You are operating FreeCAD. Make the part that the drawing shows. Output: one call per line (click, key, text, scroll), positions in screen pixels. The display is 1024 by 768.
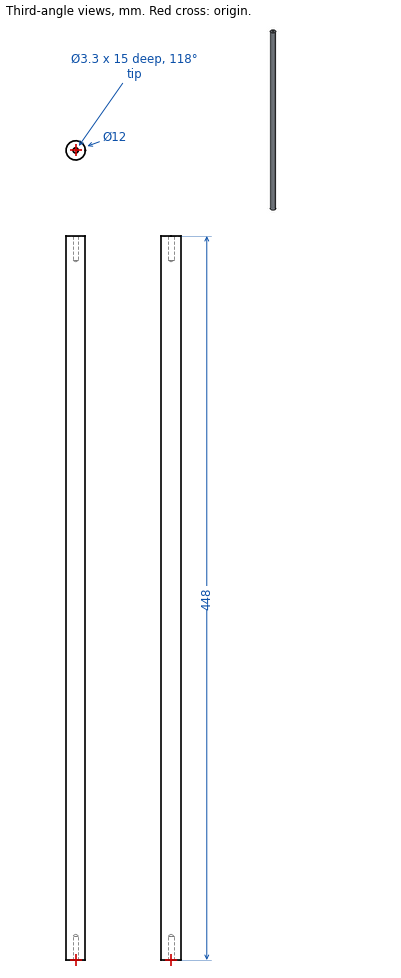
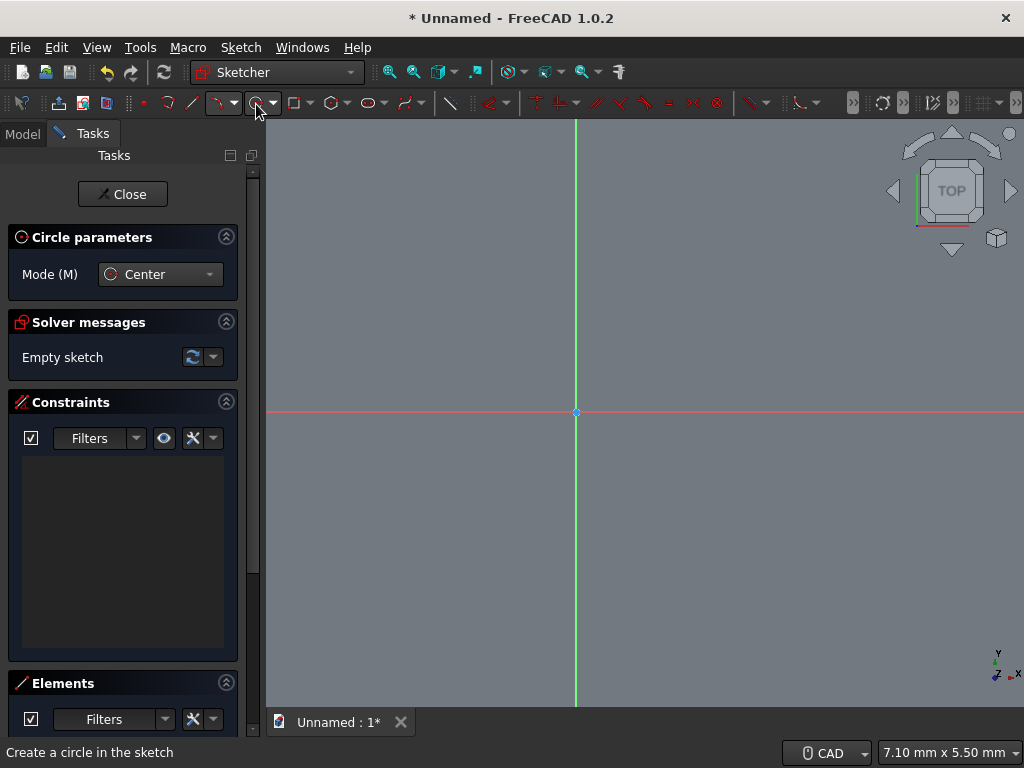
click(576, 412)
move(701, 288)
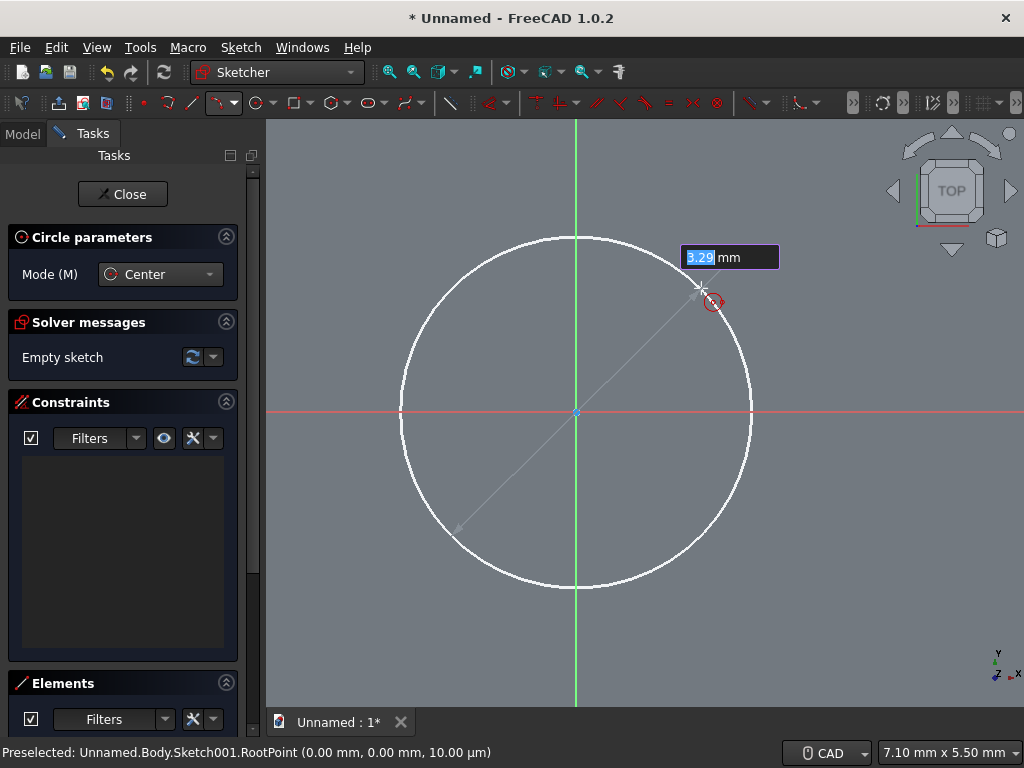
text(3.3)
key(Return)
key(Escape)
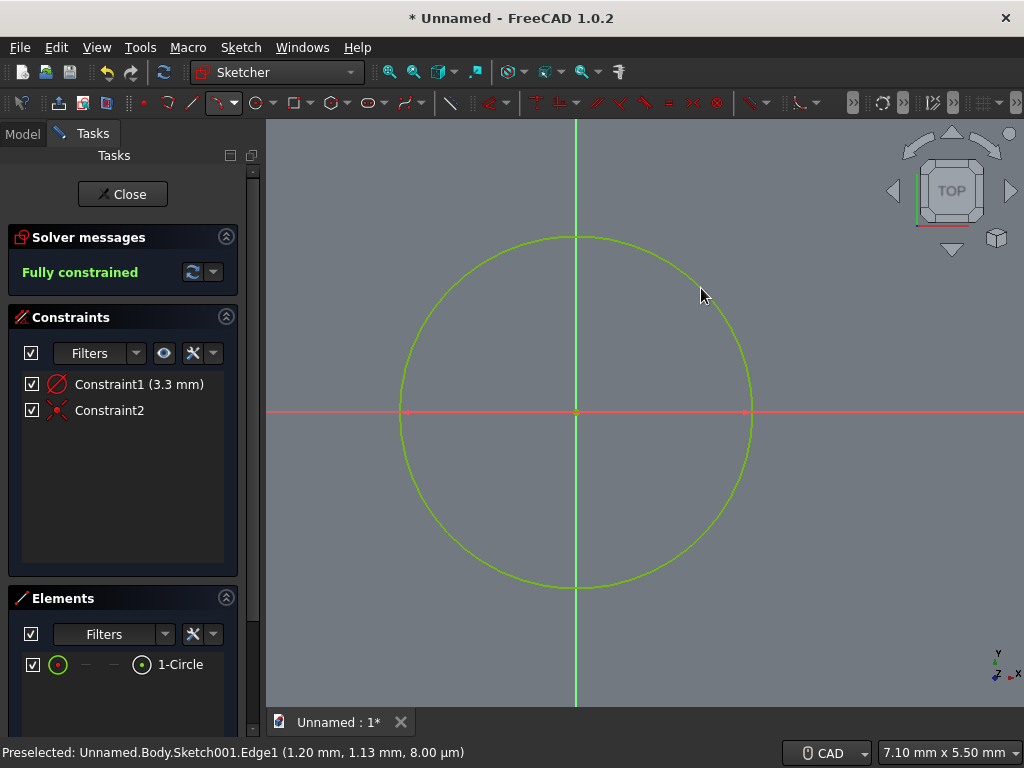
click(123, 194)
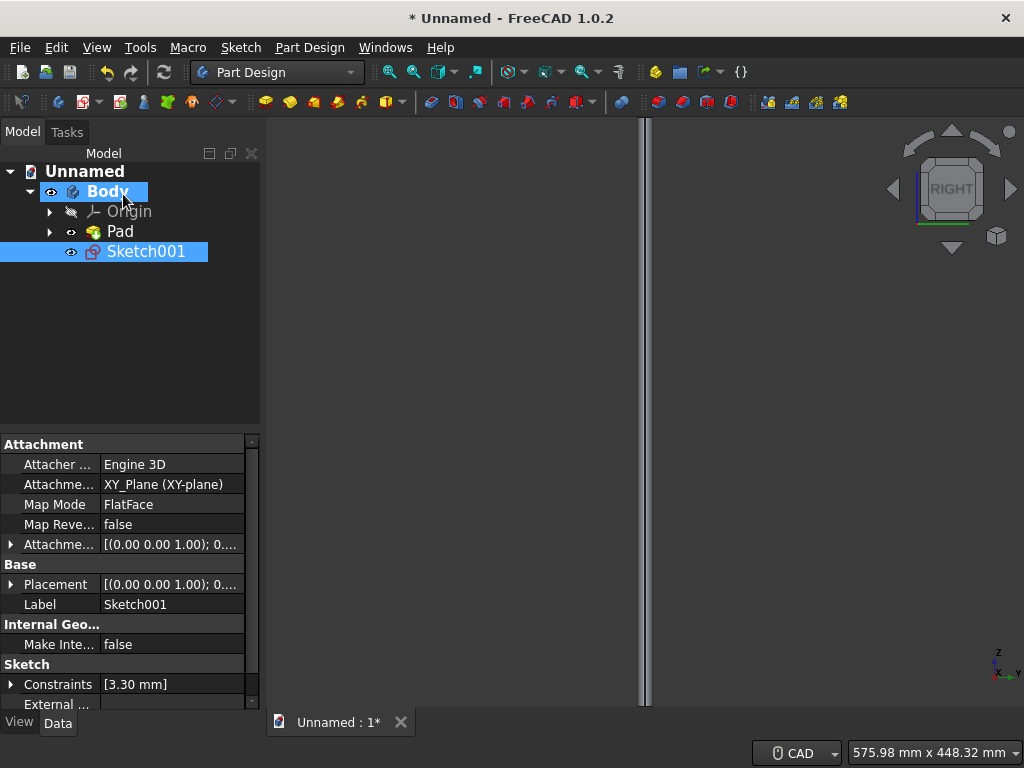
click(456, 102)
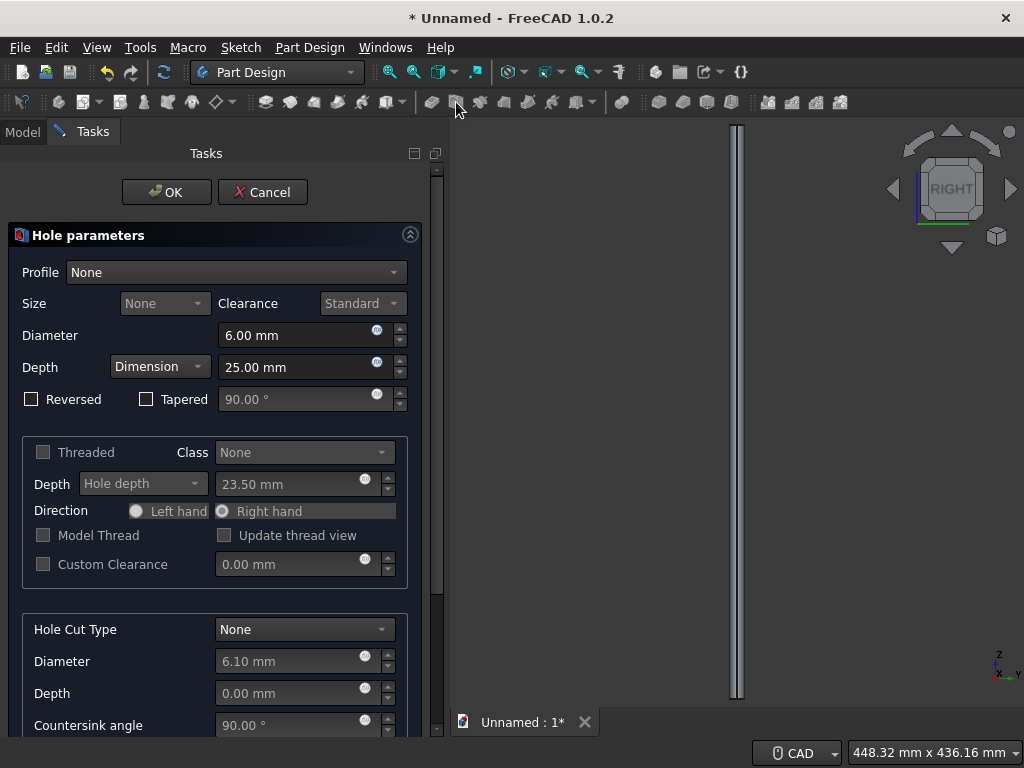
triple_click(305, 335)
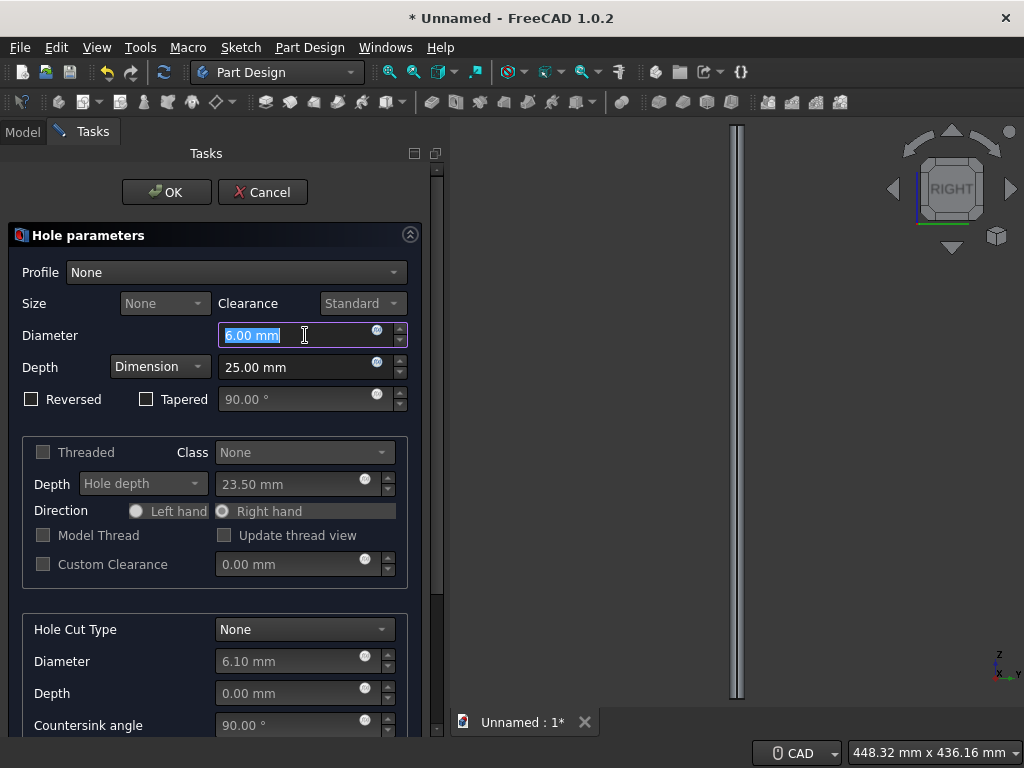
text(3.3)
key(Tab)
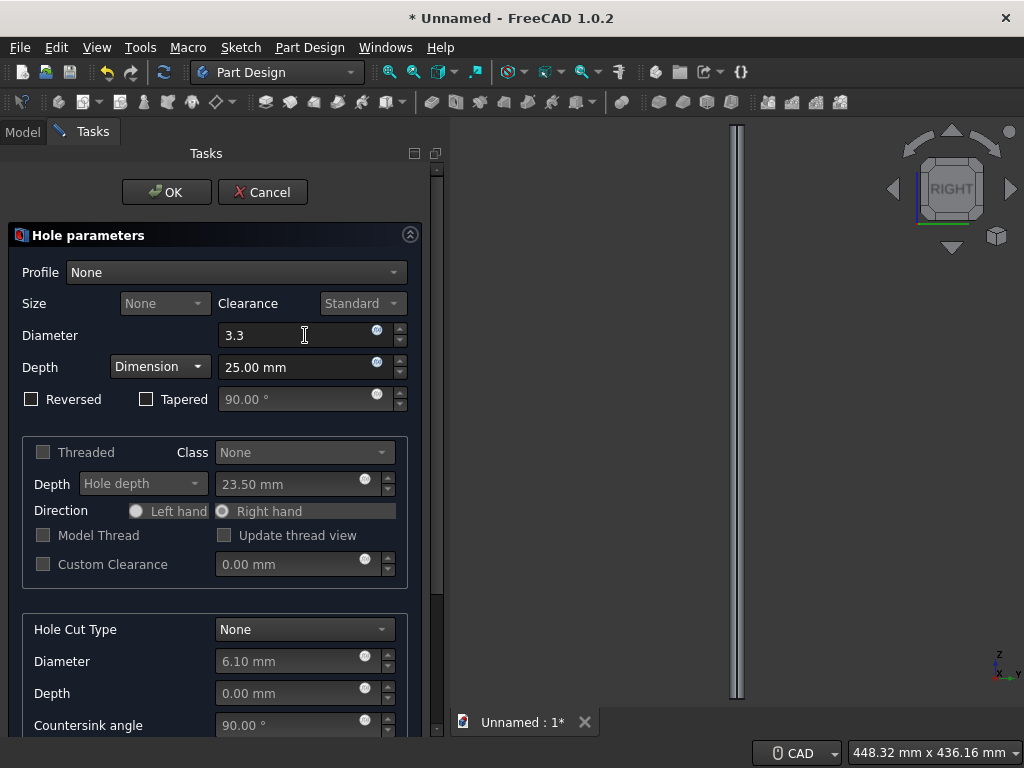
triple_click(305, 367)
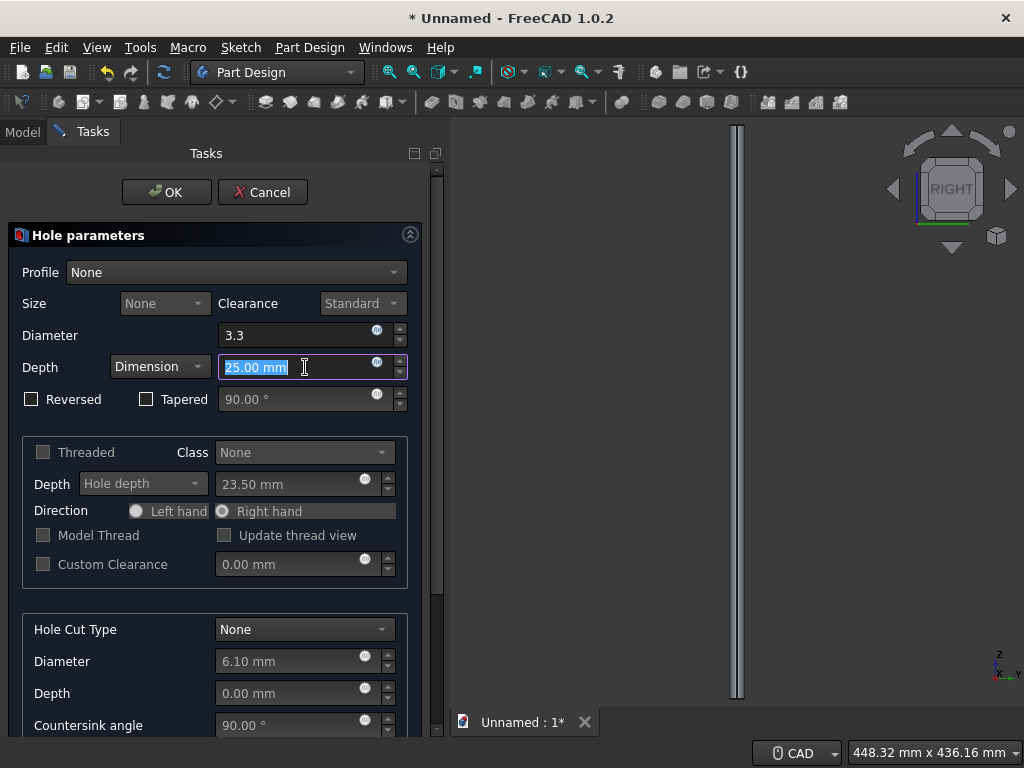
text(15)
key(Tab)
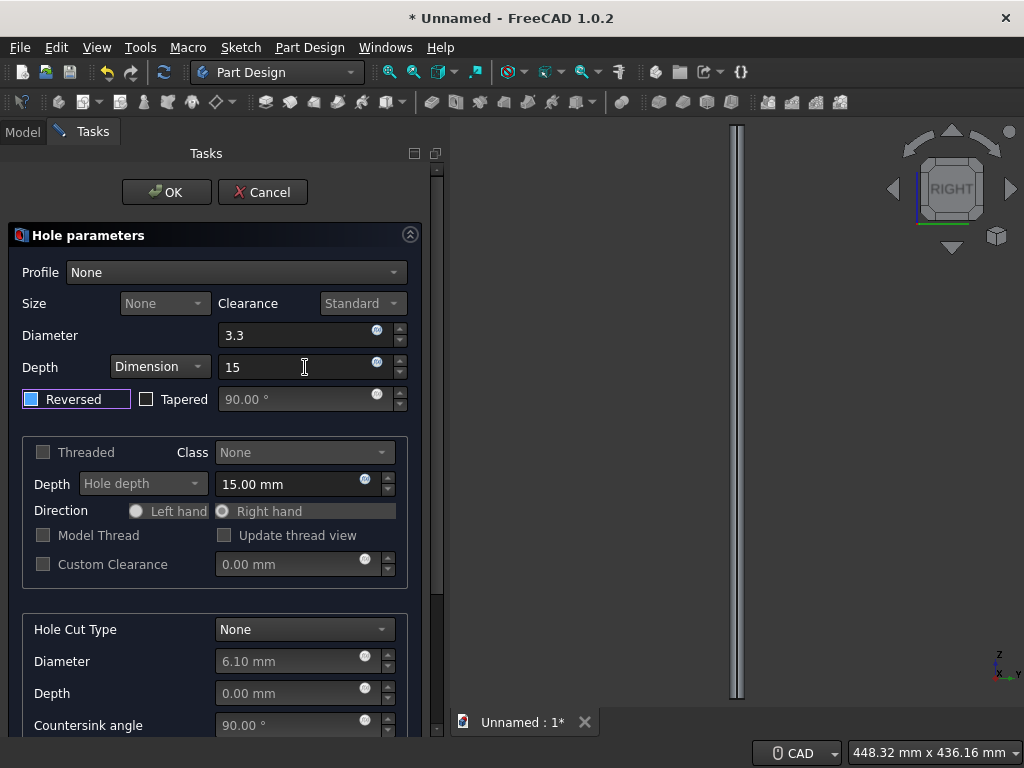
click(30, 399)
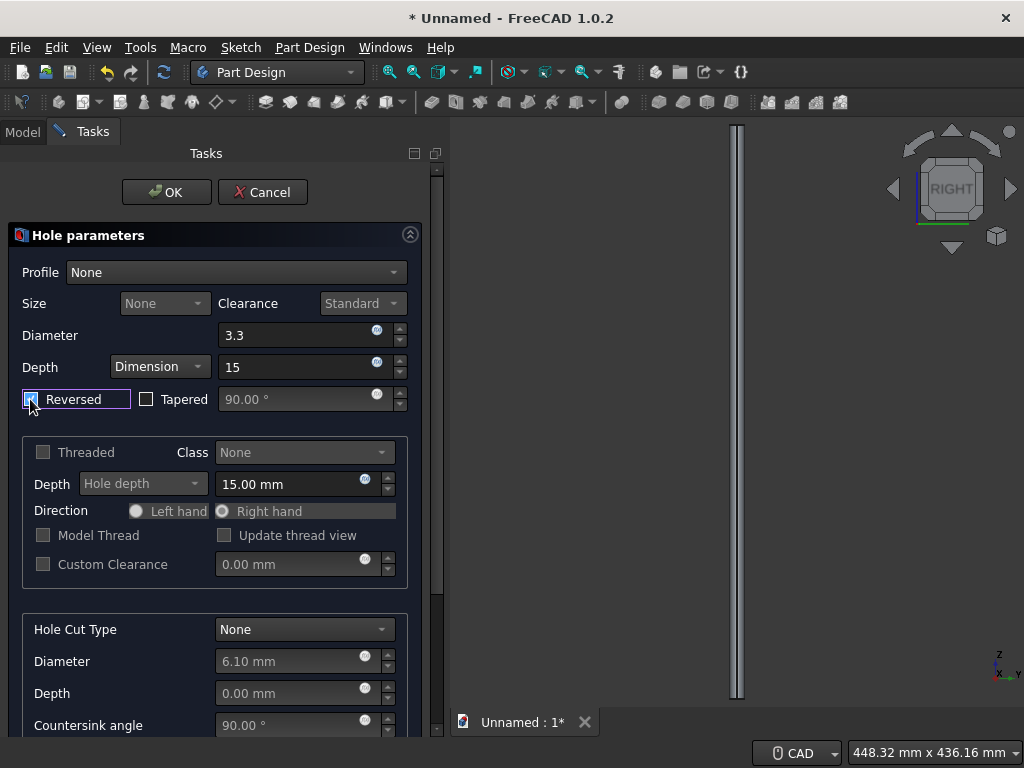
click(167, 192)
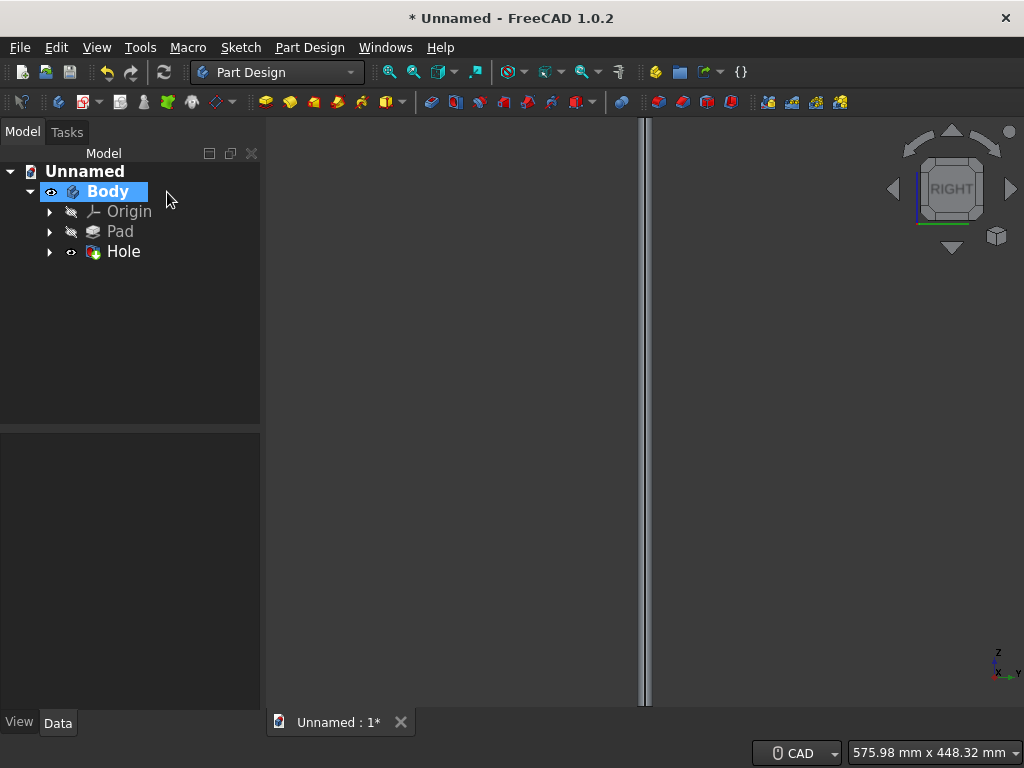
click(390, 72)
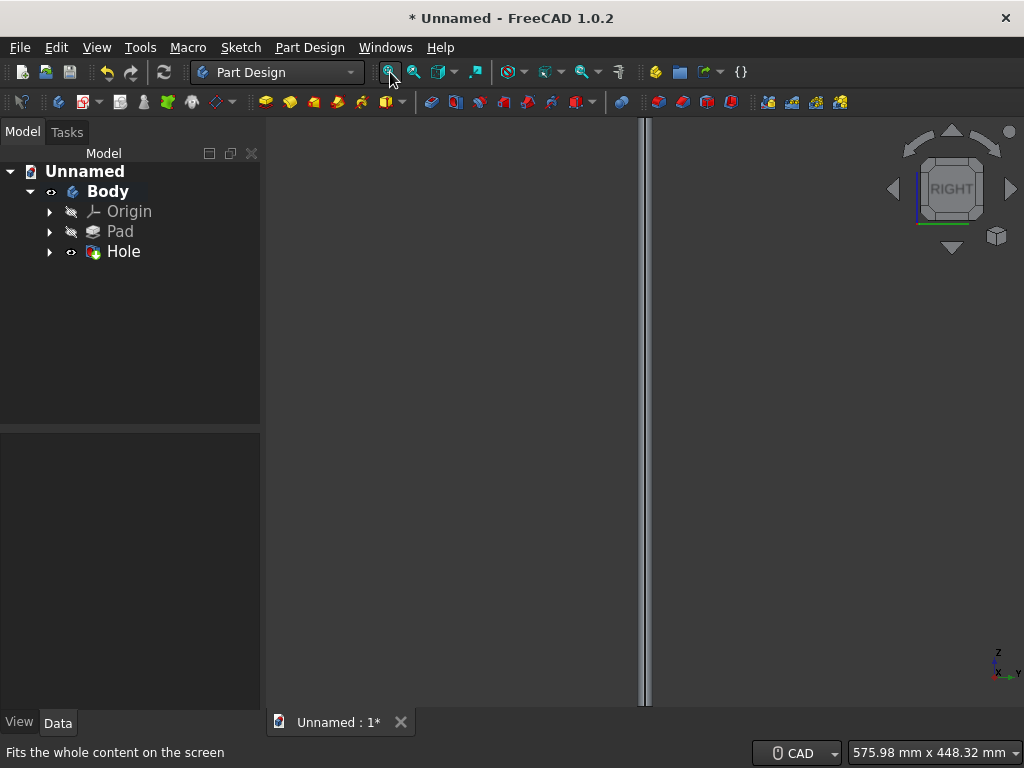
key(0)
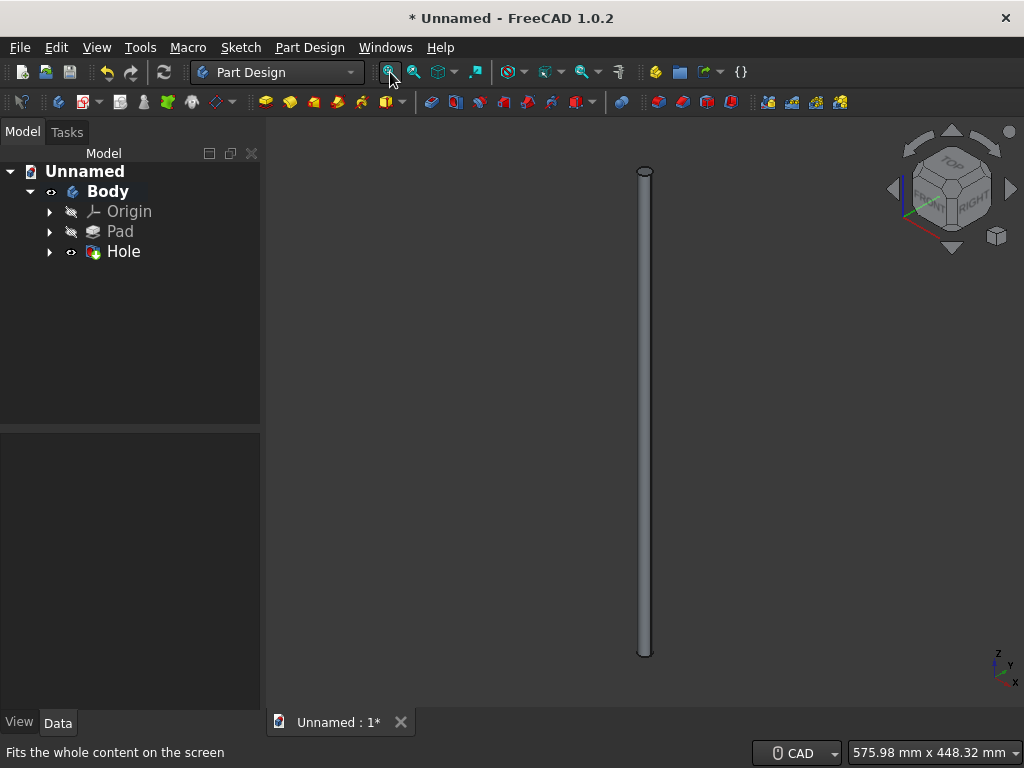
key(2)